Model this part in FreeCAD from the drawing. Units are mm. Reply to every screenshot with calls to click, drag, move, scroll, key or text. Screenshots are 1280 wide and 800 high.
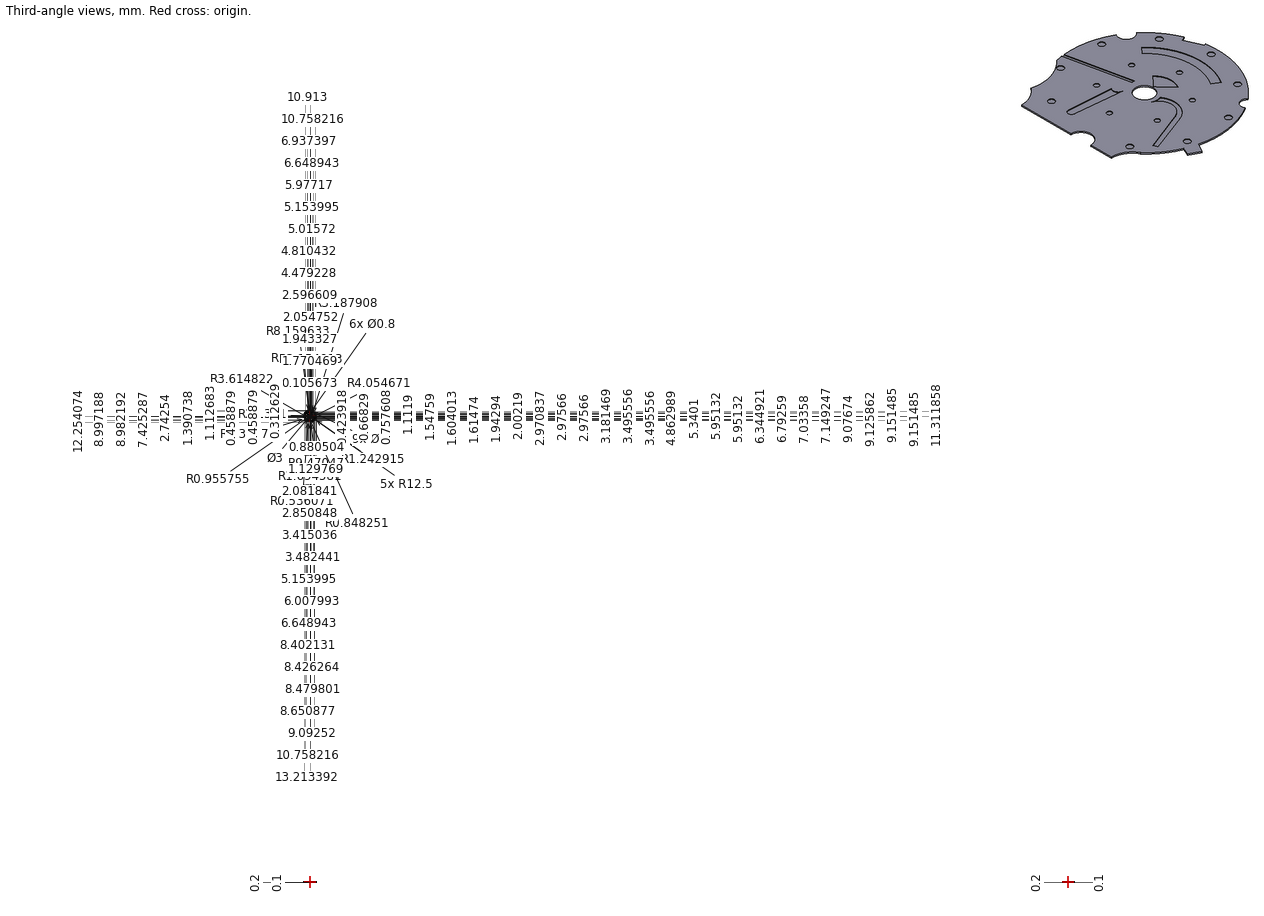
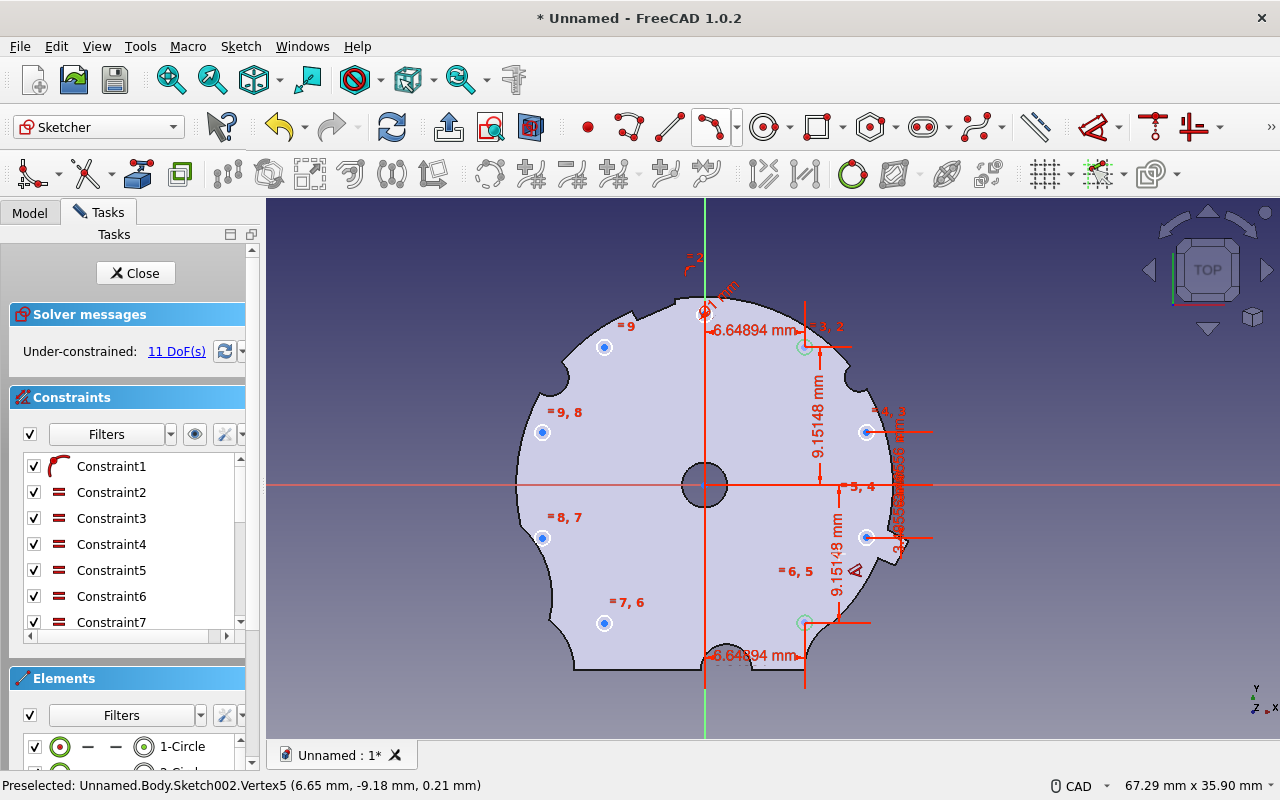
click(604, 623)
click(655, 657)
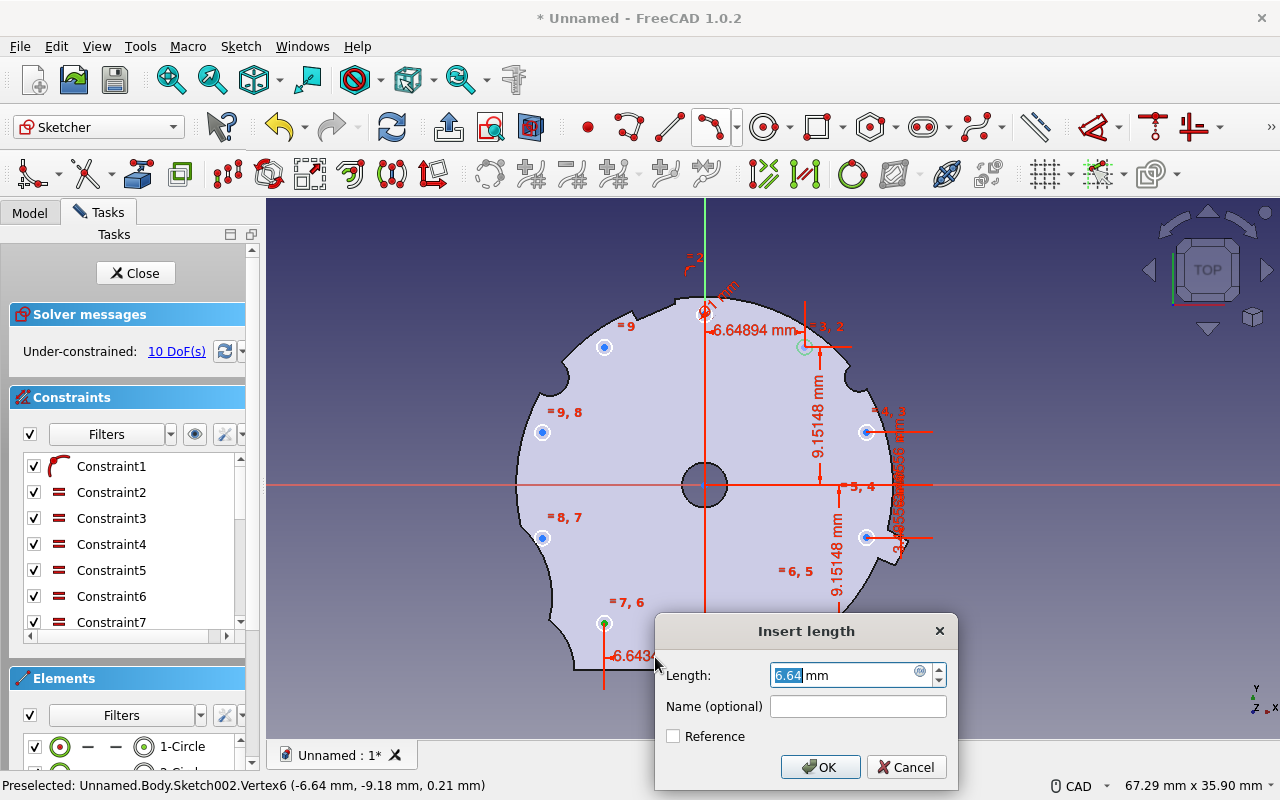
text(6.648943)
key(Return)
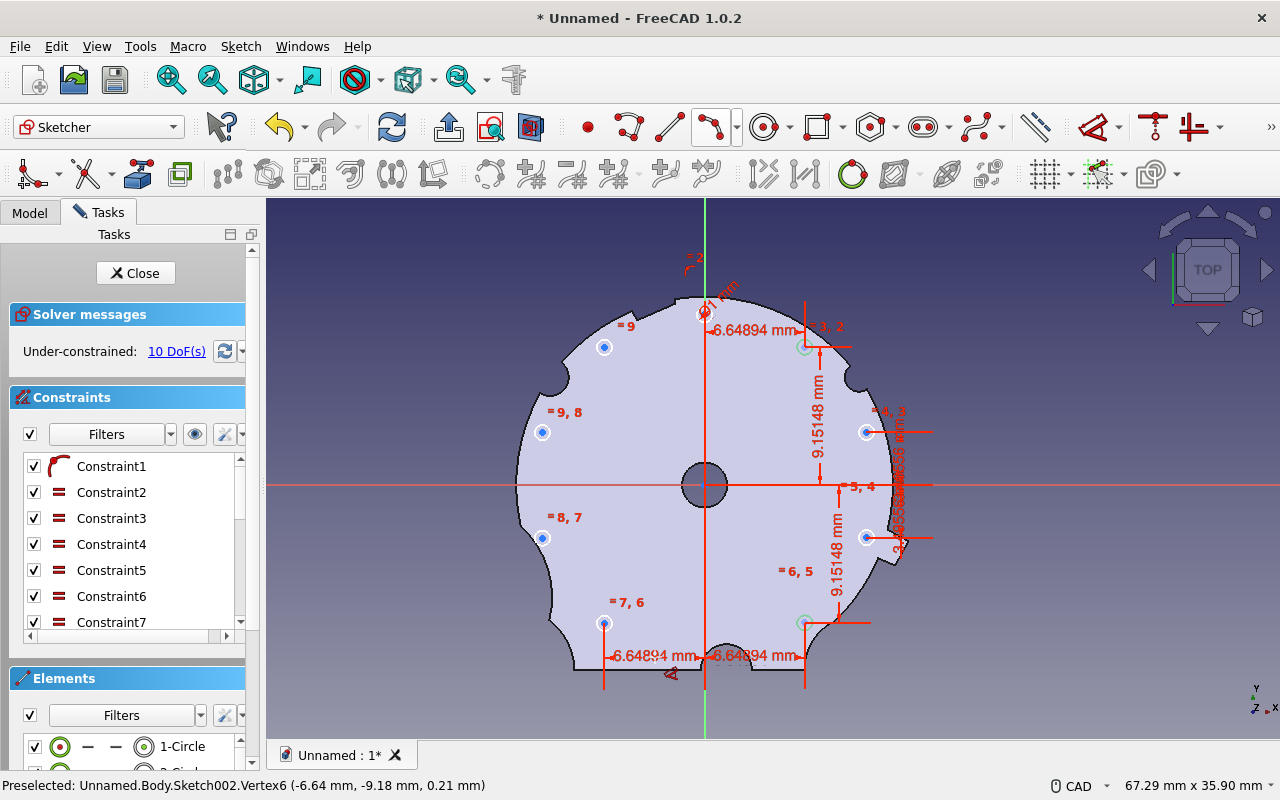
click(604, 623)
click(570, 554)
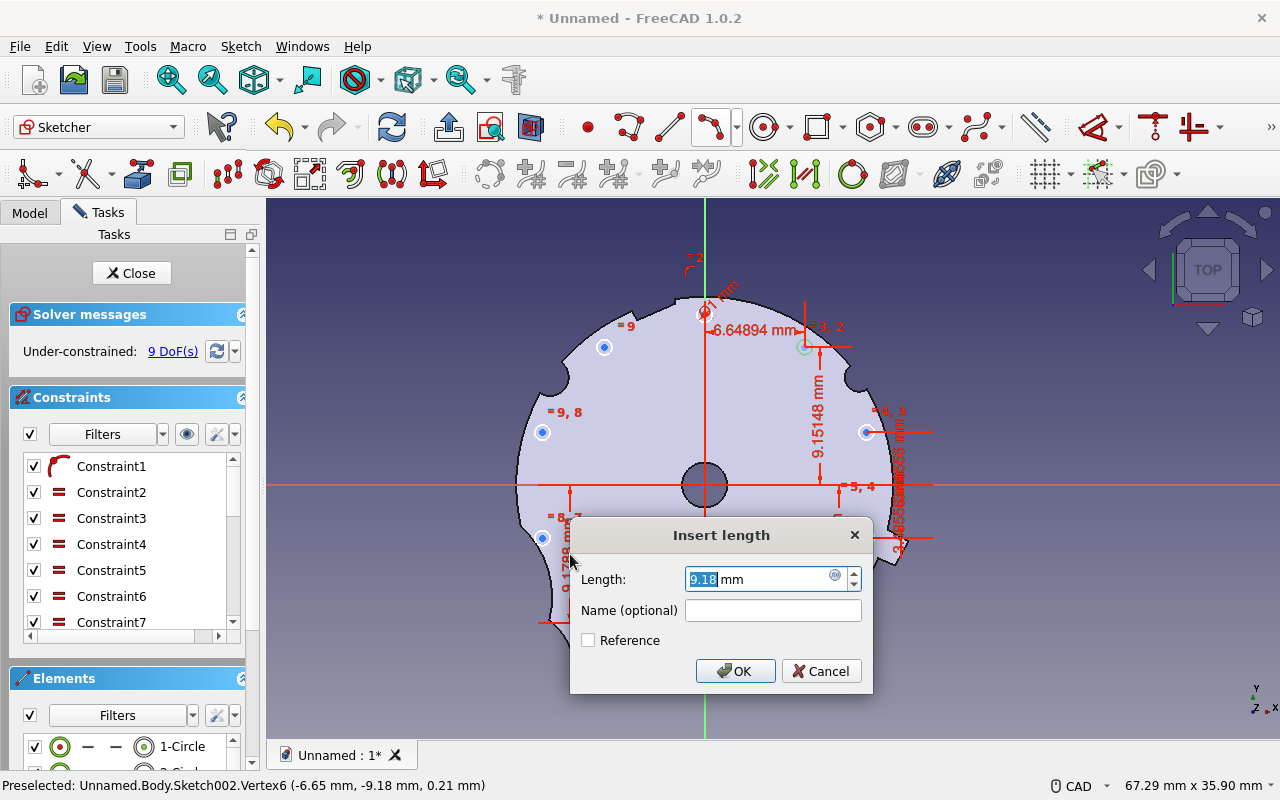
text(9.151485)
key(Return)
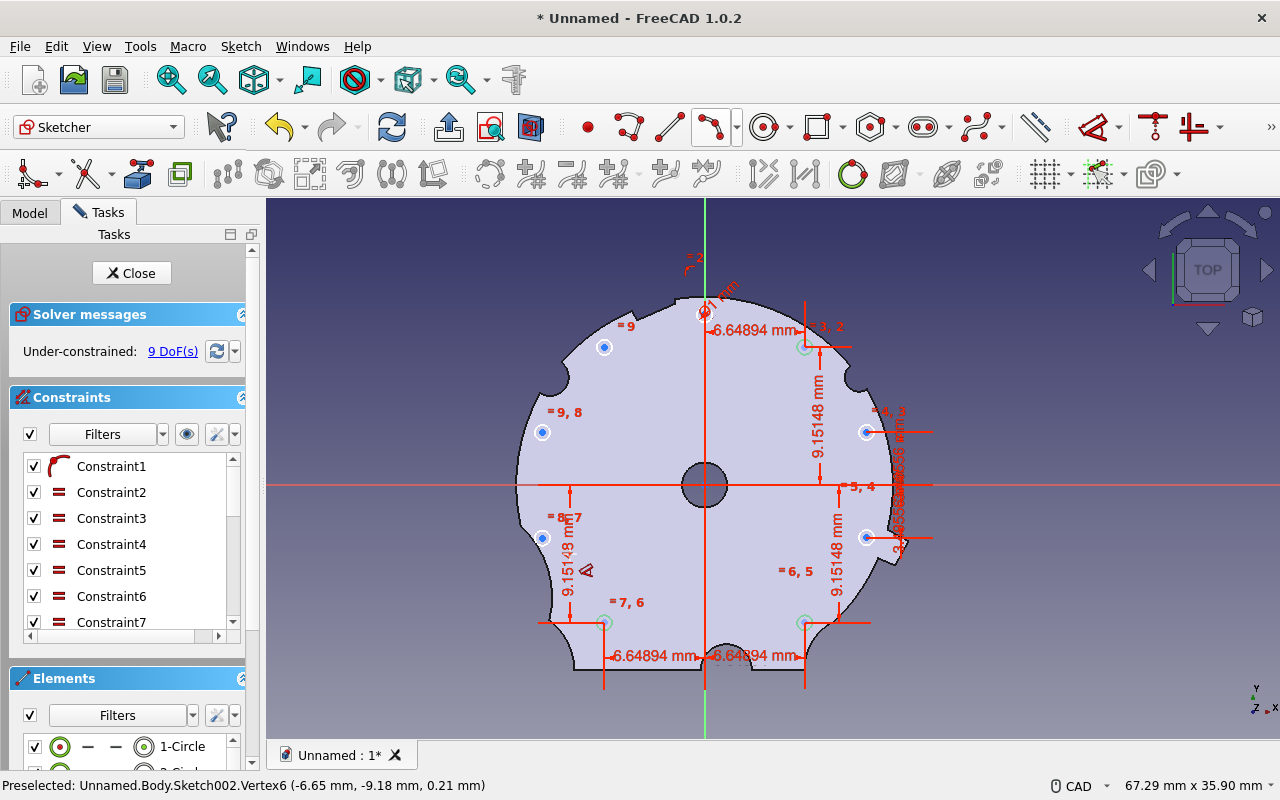
click(542, 538)
click(508, 512)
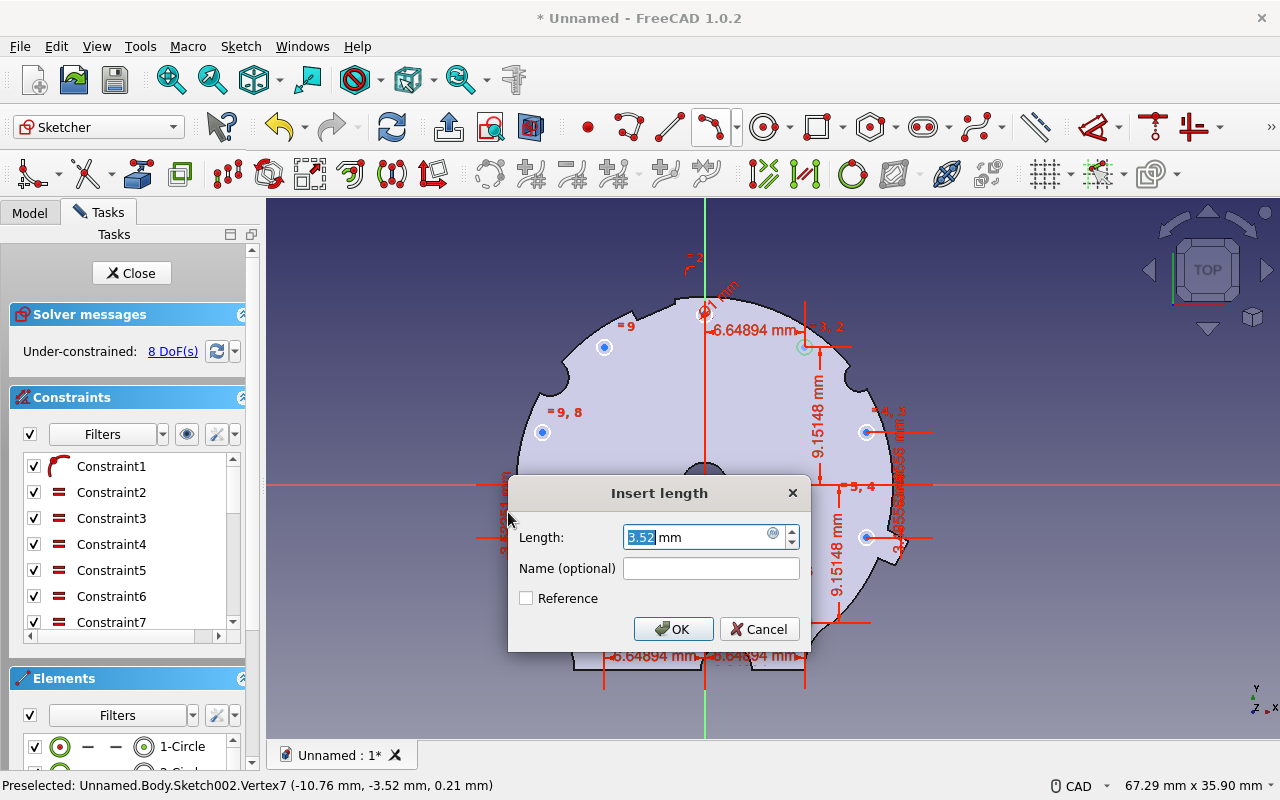
text(3.495556)
key(Return)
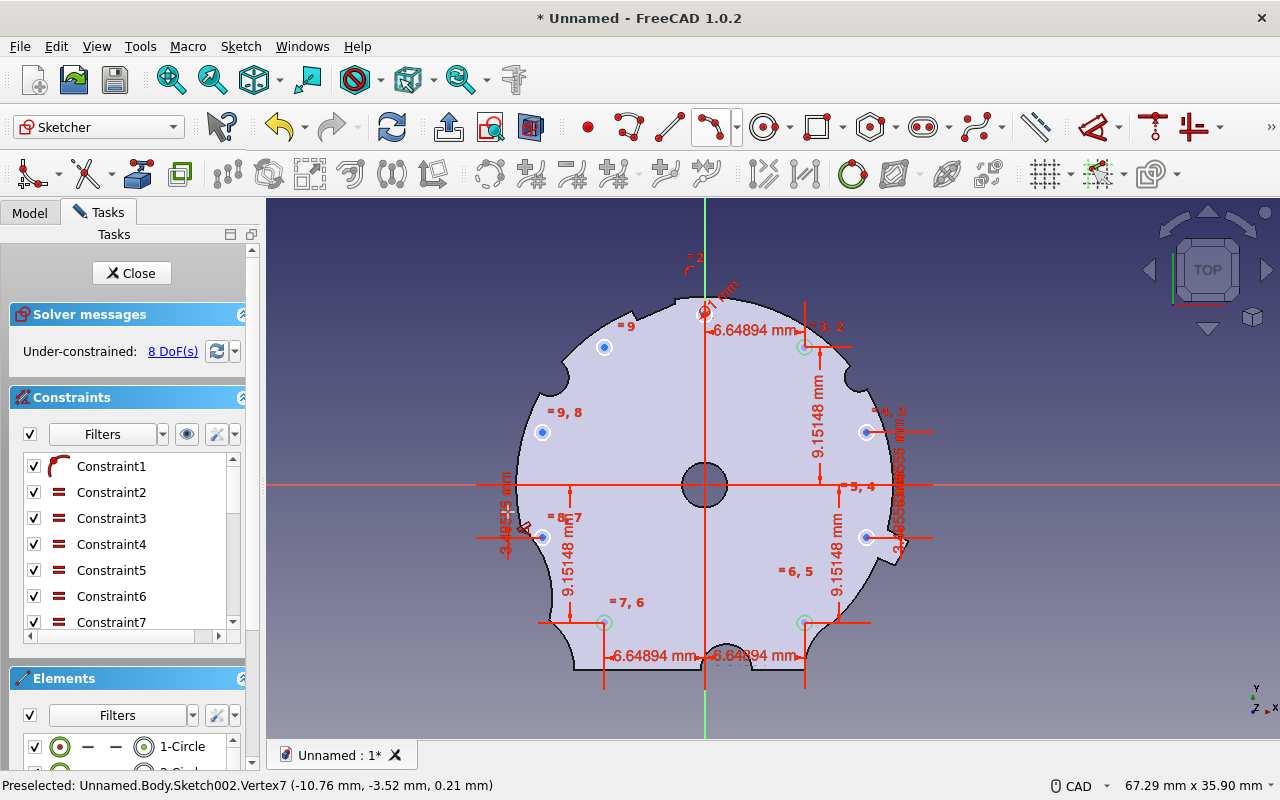
click(542, 433)
click(508, 459)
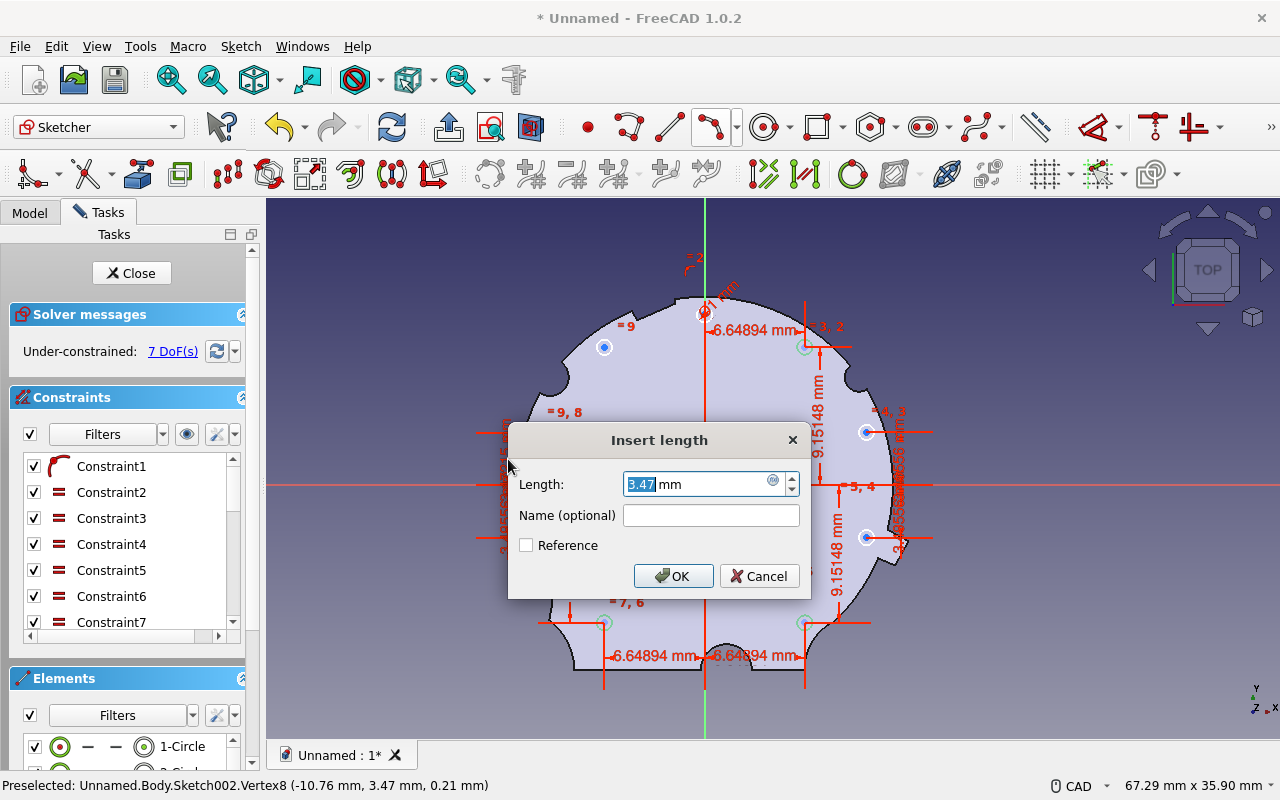
text(3.495556)
key(Return)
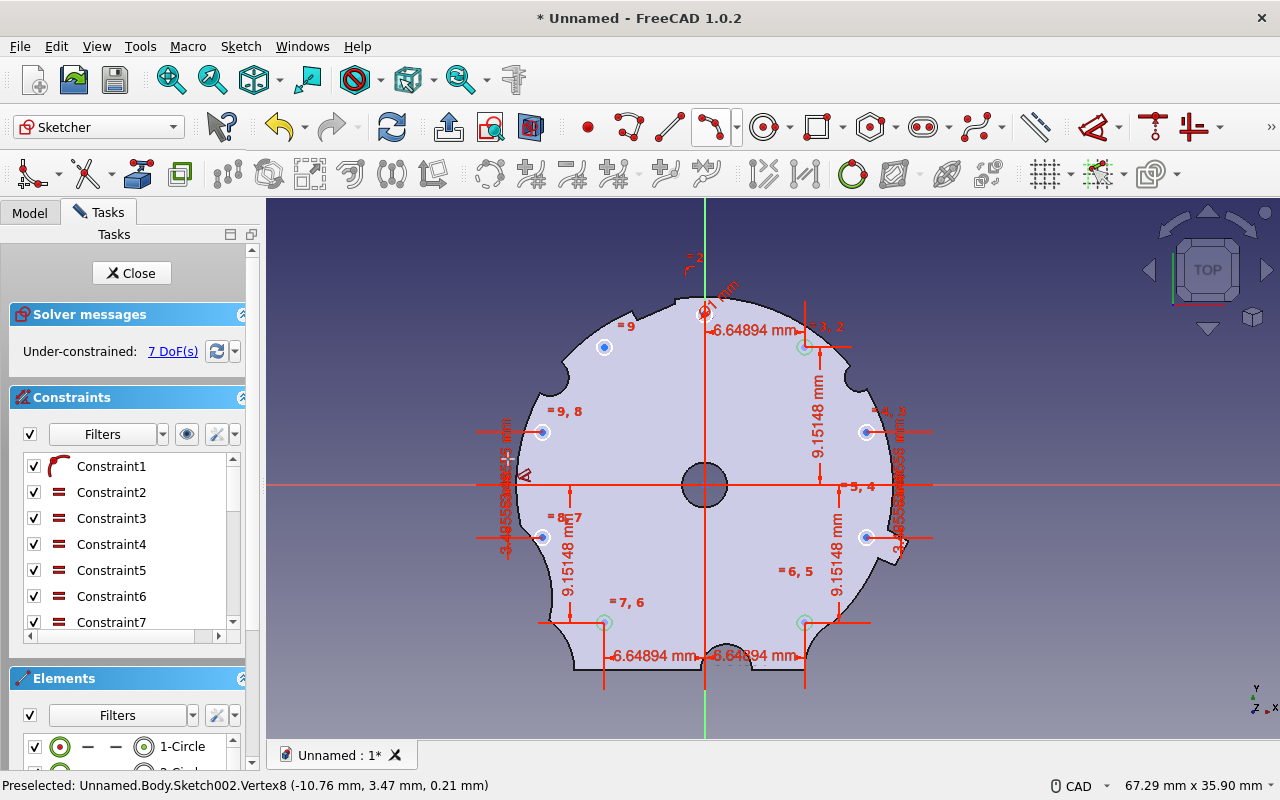
click(604, 347)
click(632, 313)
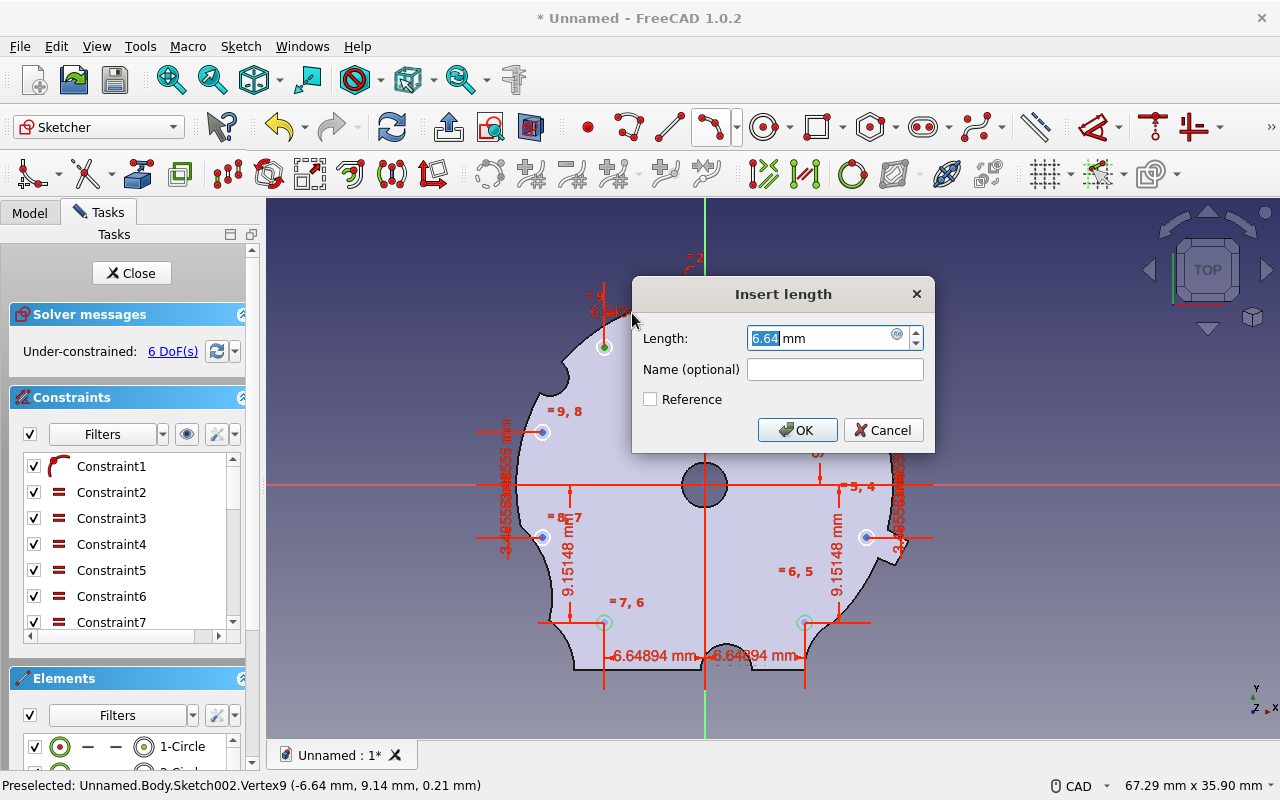
text(6.648943)
key(Return)